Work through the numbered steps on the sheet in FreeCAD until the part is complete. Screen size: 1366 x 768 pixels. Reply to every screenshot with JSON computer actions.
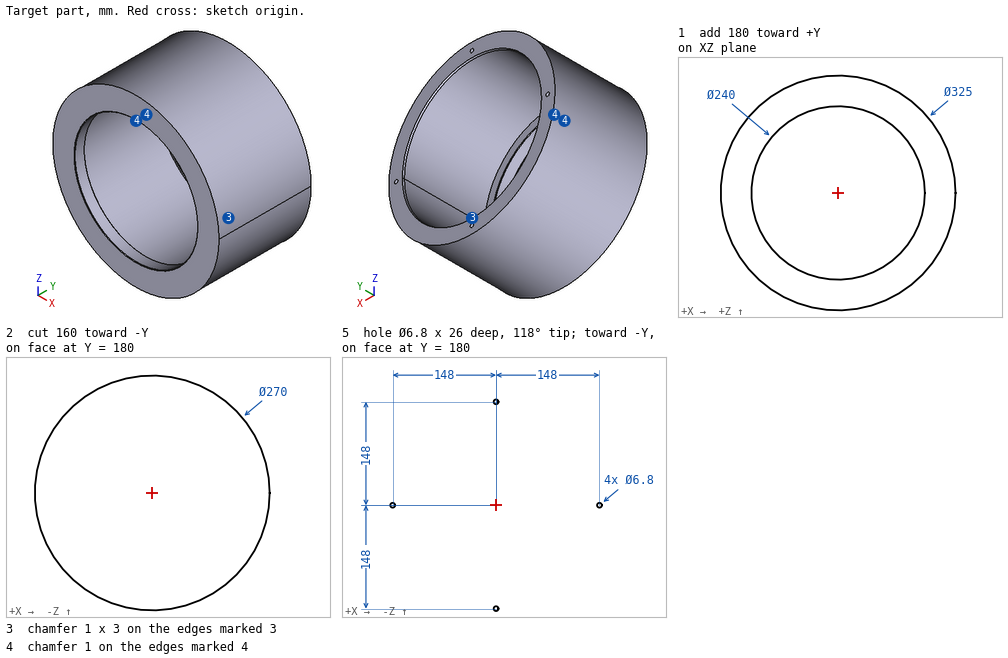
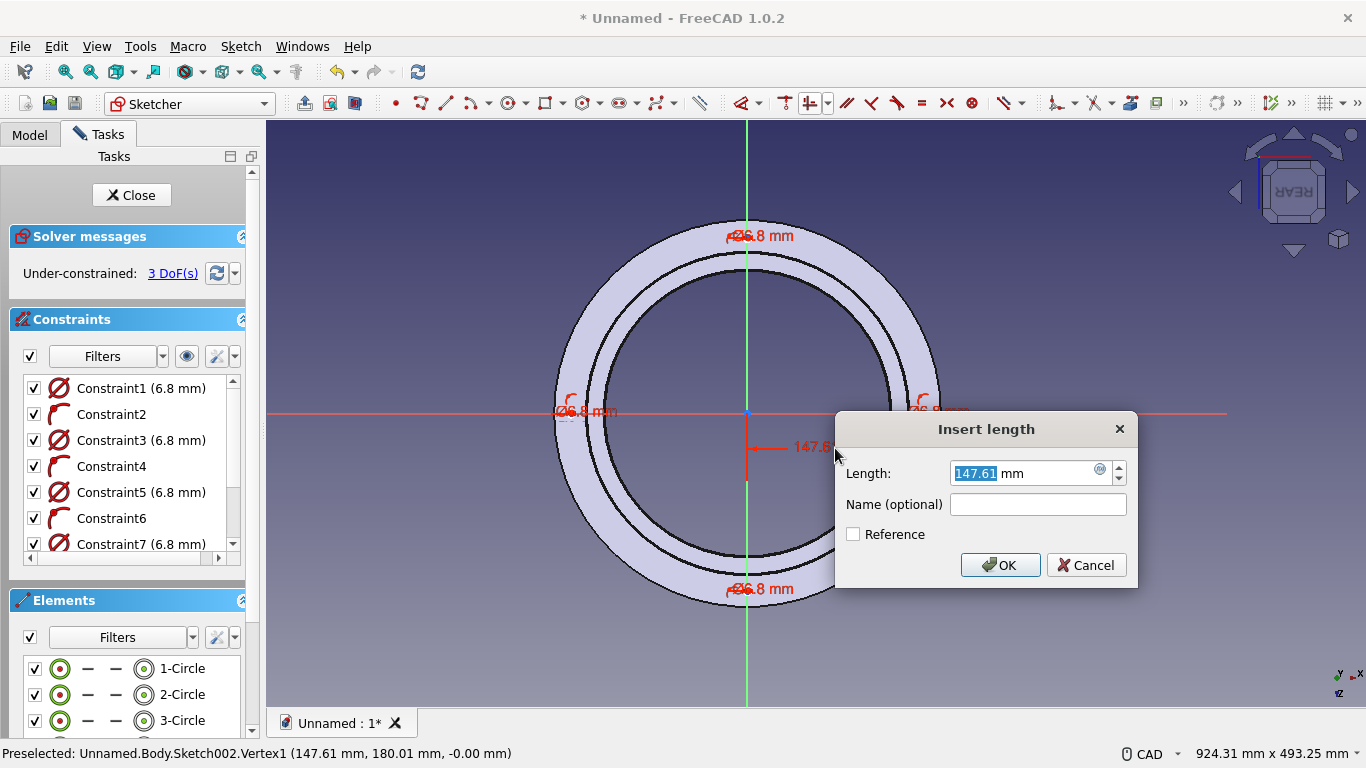
{"action": "type", "text": "148"}
{"action": "key", "text": "Return"}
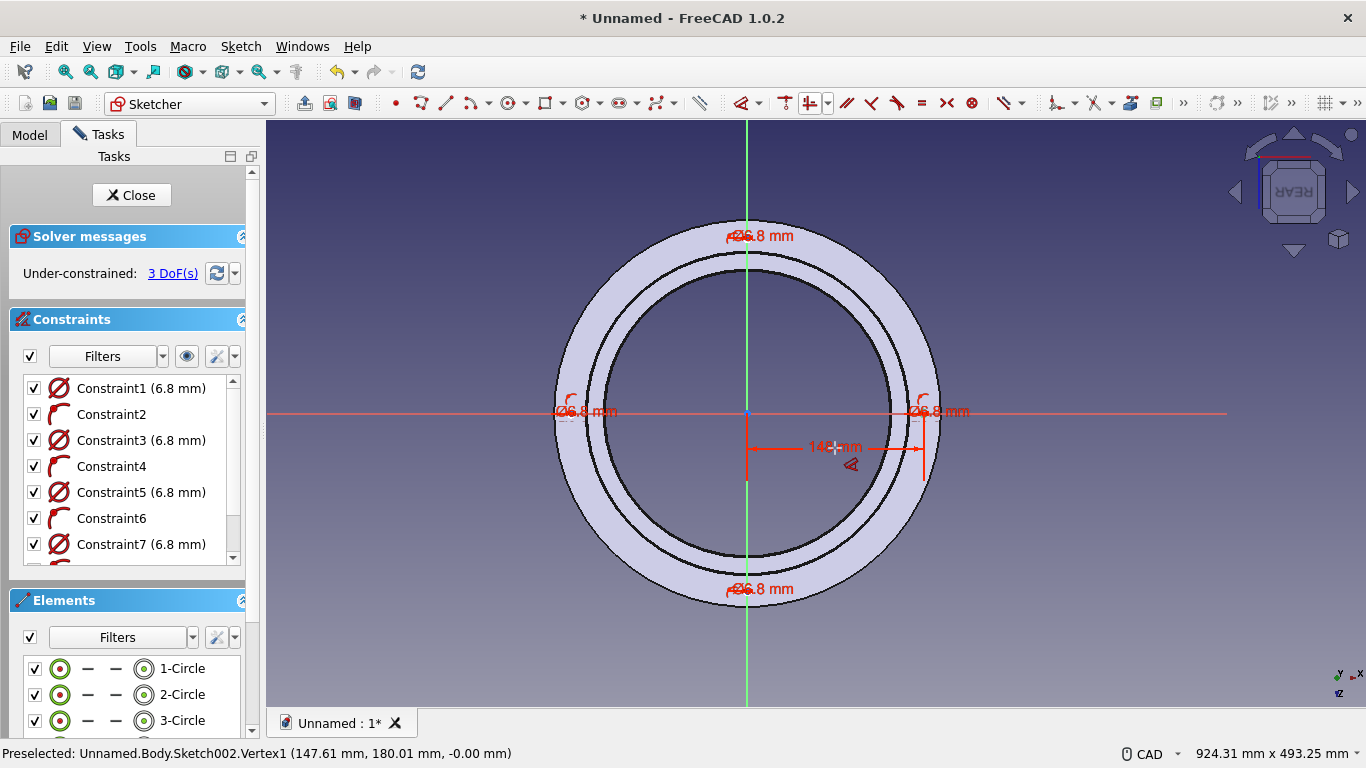
{"action": "left_click", "coordinate": [747, 591]}
{"action": "left_click", "coordinate": [781, 502]}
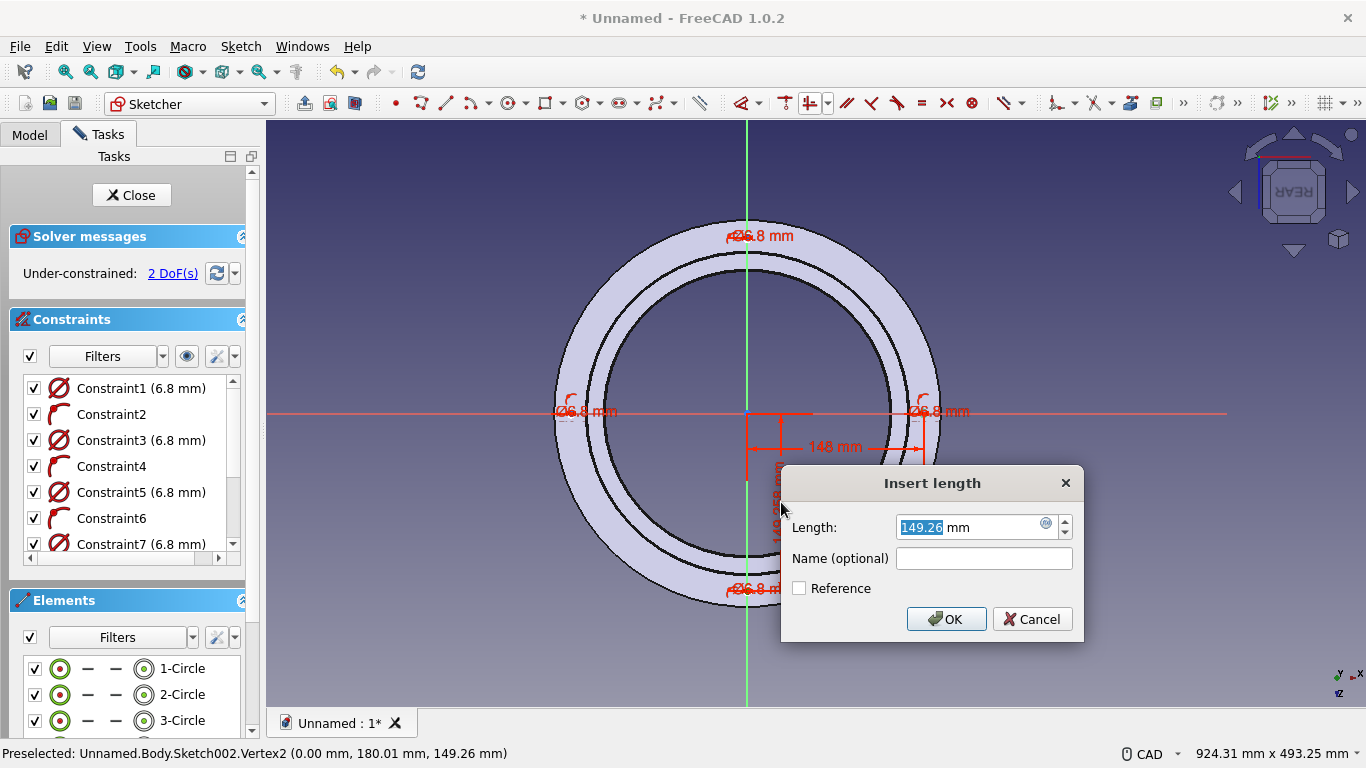
{"action": "type", "text": "148"}
{"action": "key", "text": "Return"}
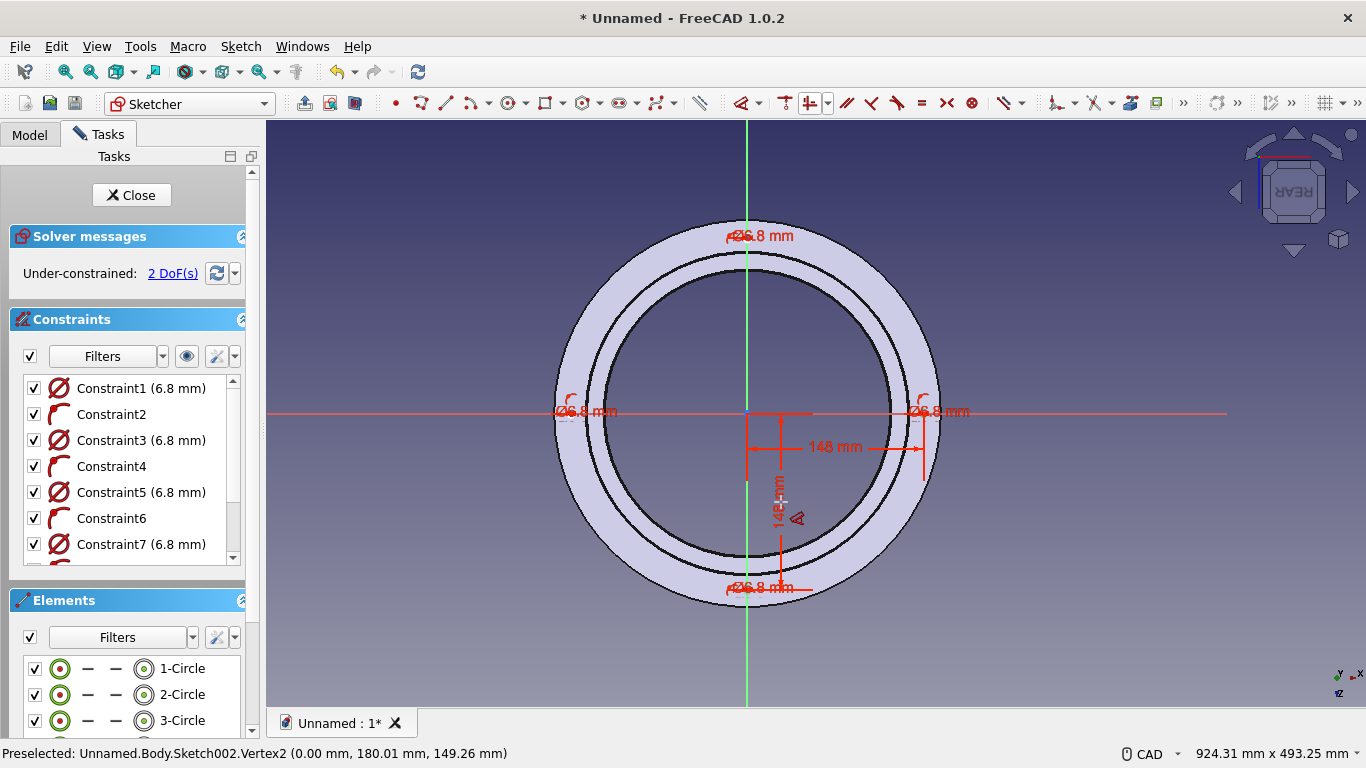
{"action": "left_click", "coordinate": [571, 414]}
{"action": "left_click", "coordinate": [659, 448]}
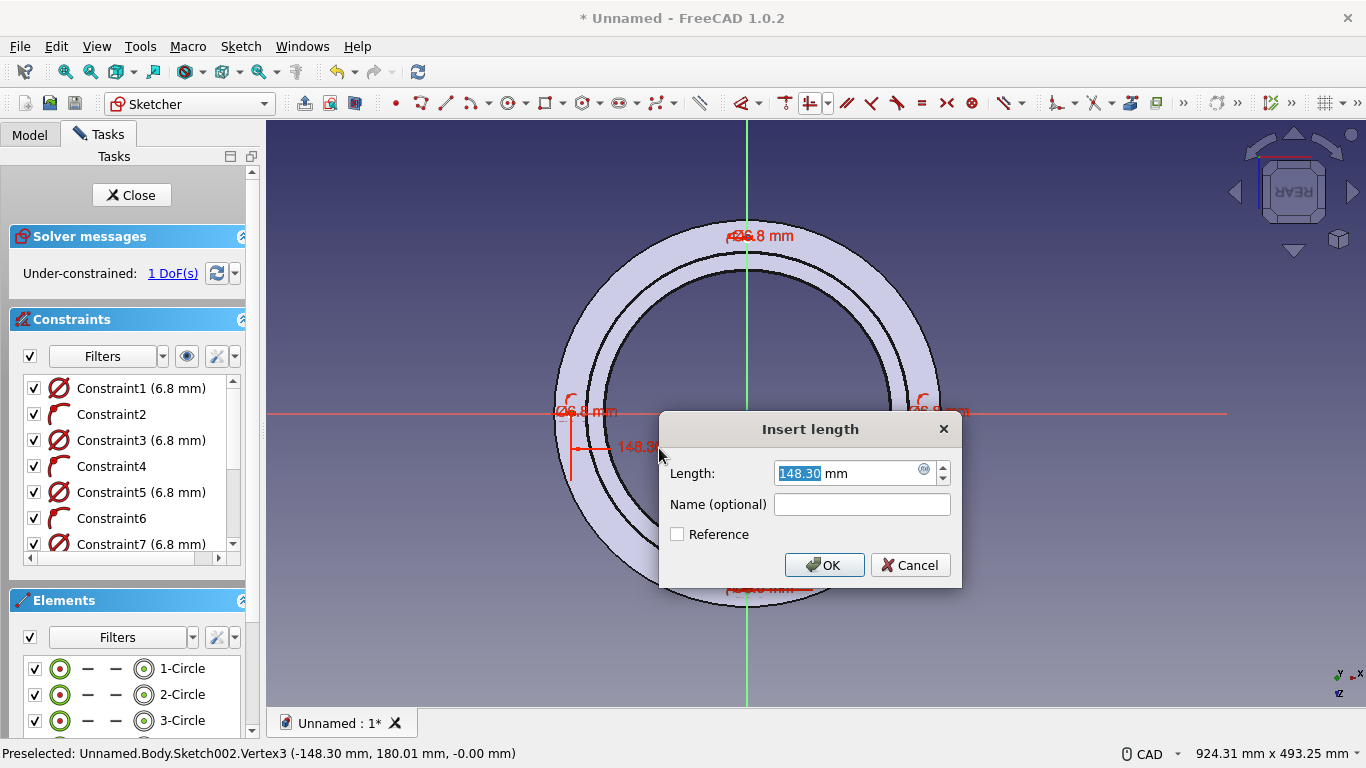
{"action": "type", "text": "148"}
{"action": "key", "text": "Return"}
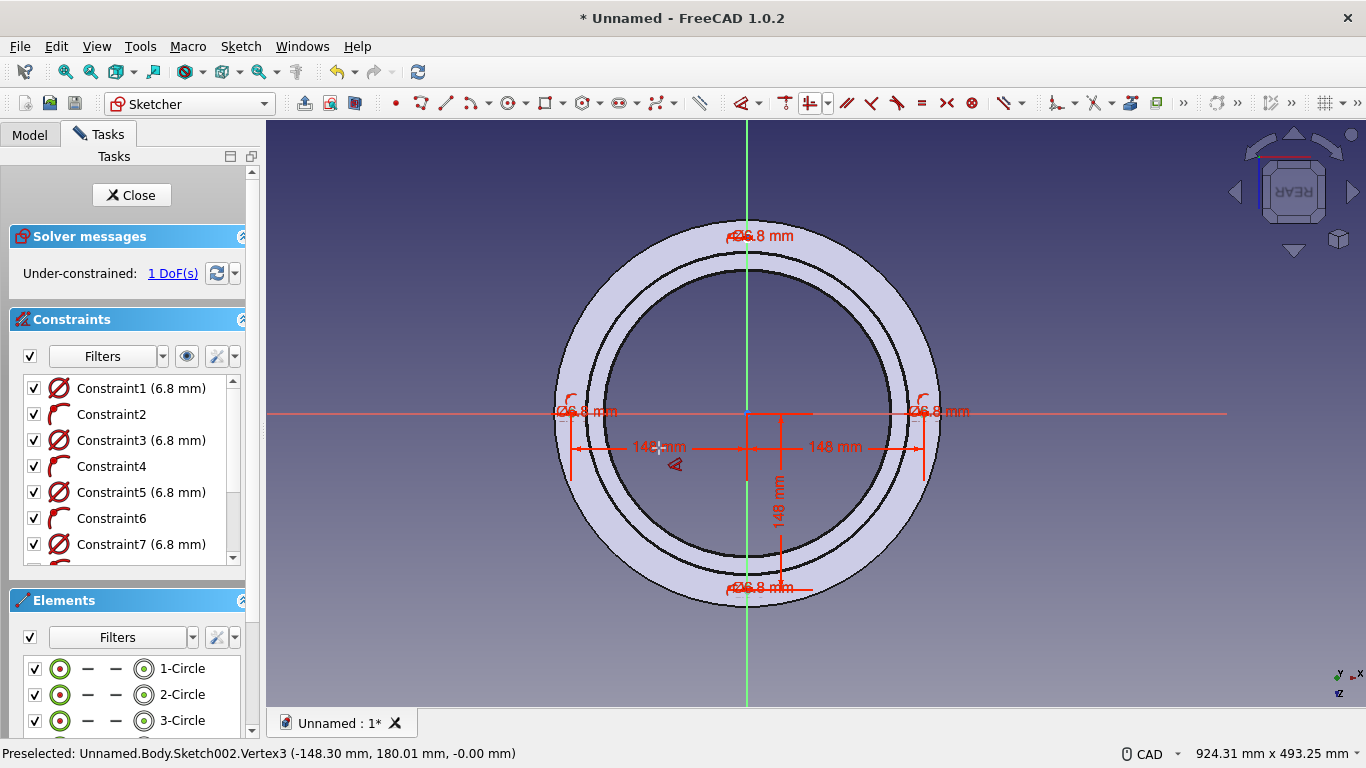
{"action": "left_click", "coordinate": [747, 238]}
{"action": "left_click", "coordinate": [781, 326]}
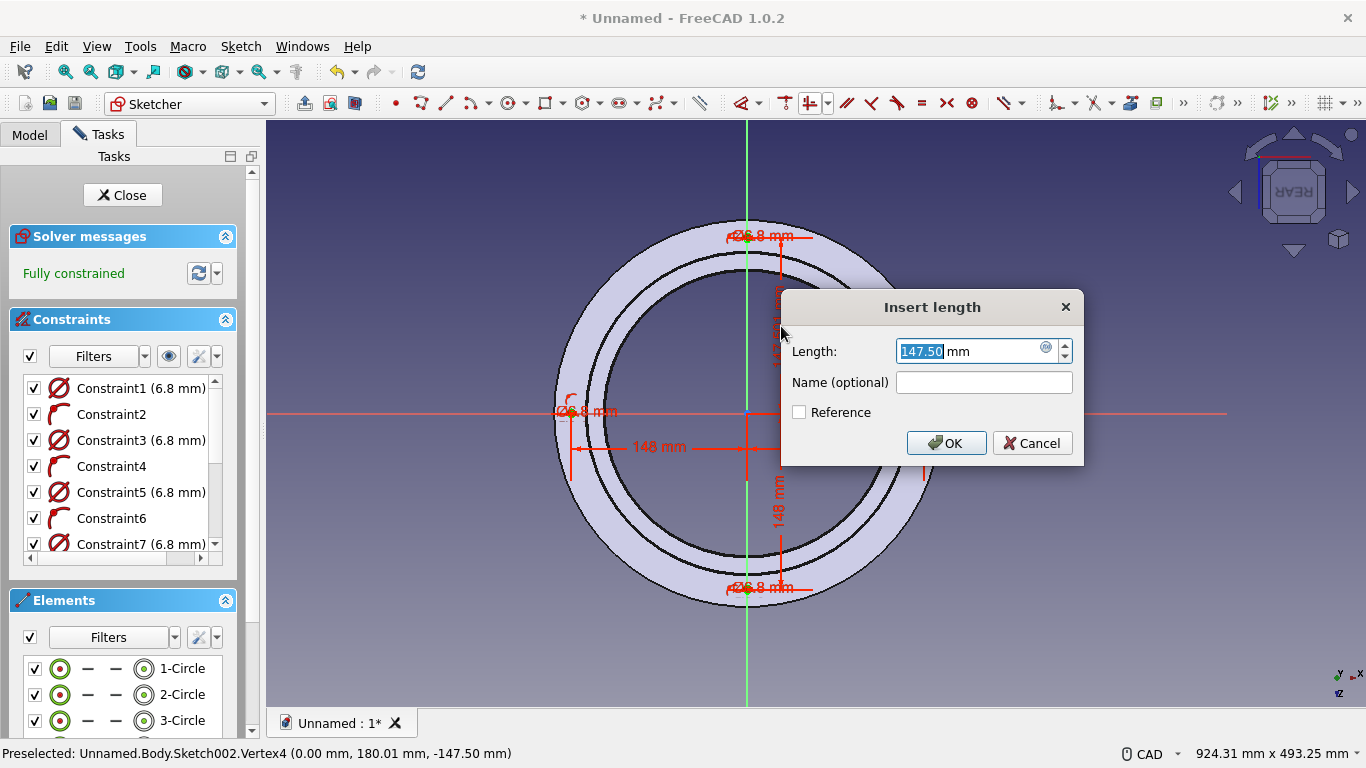
{"action": "type", "text": "148"}
{"action": "key", "text": "Return"}
{"action": "key", "text": "Escape"}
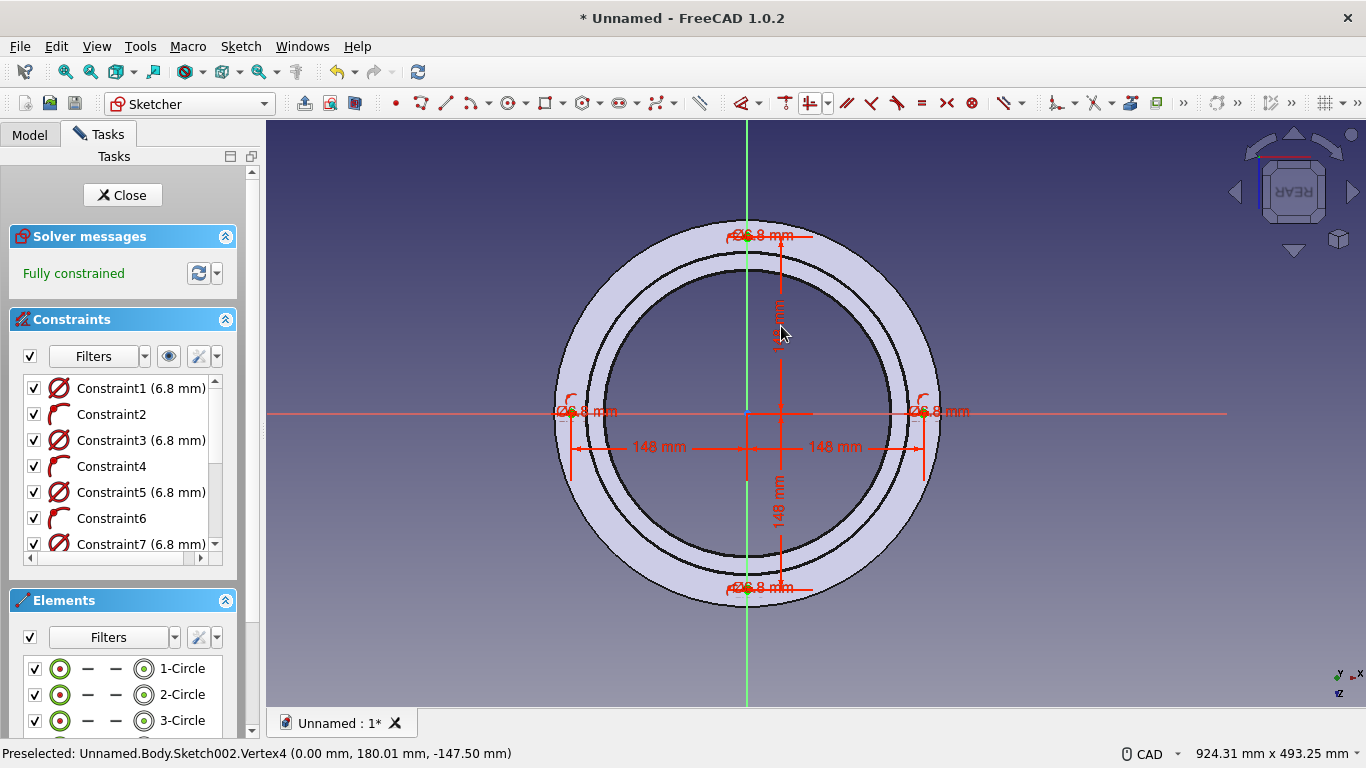
{"action": "left_click", "coordinate": [123, 195]}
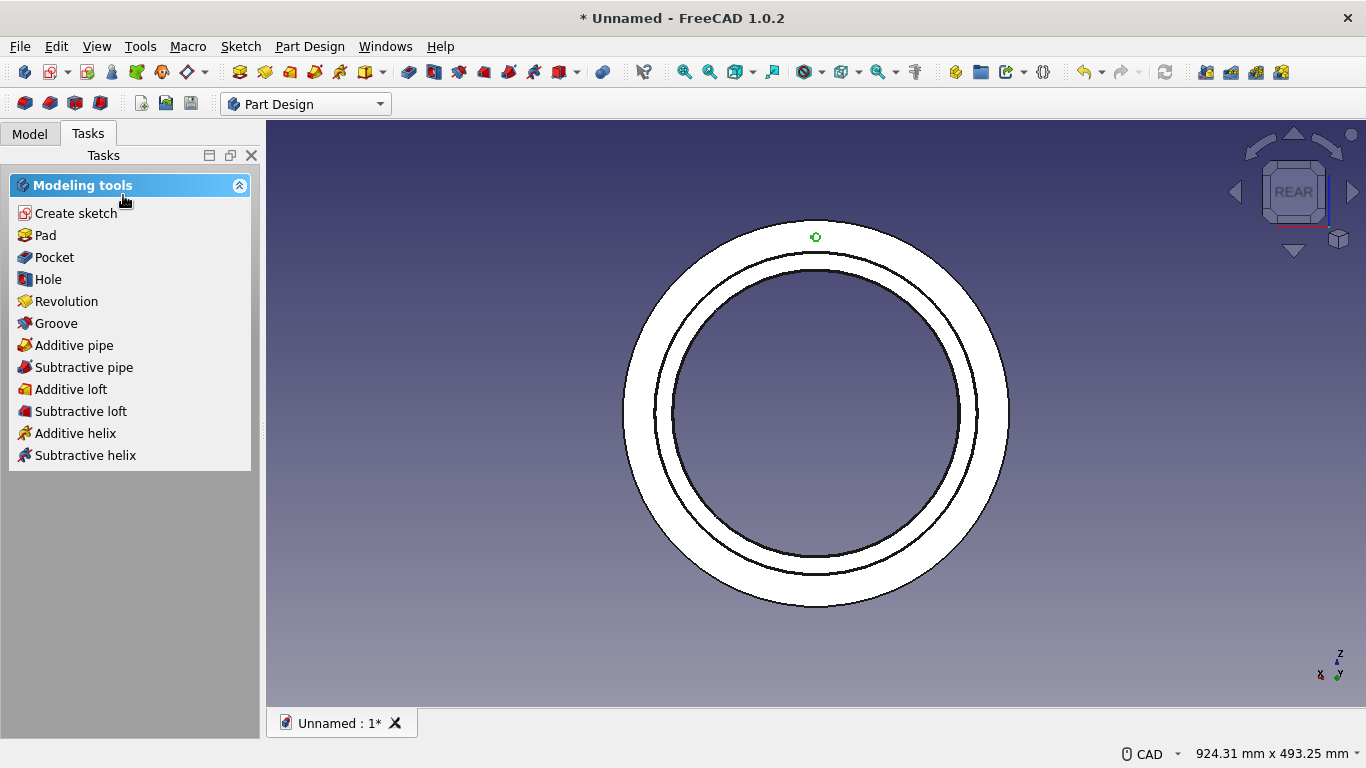
{"action": "left_click", "coordinate": [434, 72]}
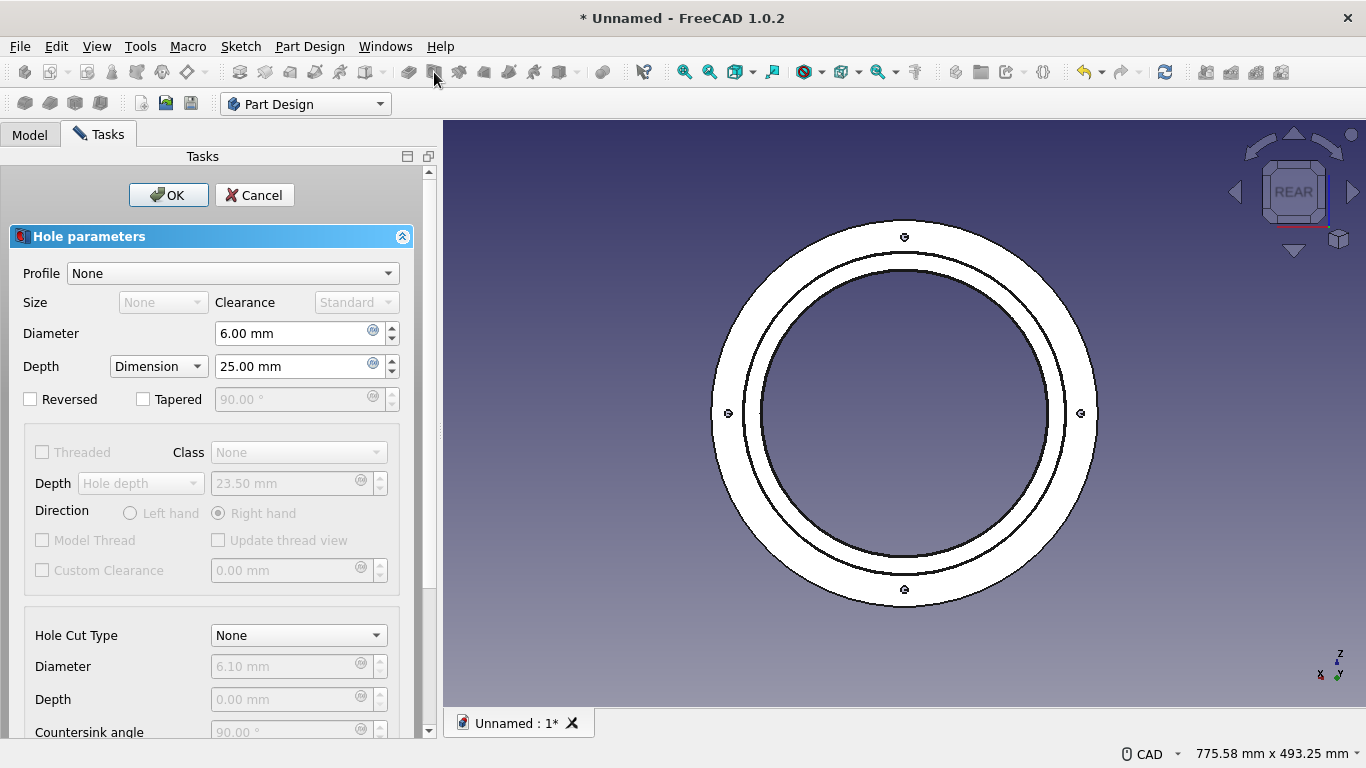
{"action": "triple_click", "coordinate": [300, 334]}